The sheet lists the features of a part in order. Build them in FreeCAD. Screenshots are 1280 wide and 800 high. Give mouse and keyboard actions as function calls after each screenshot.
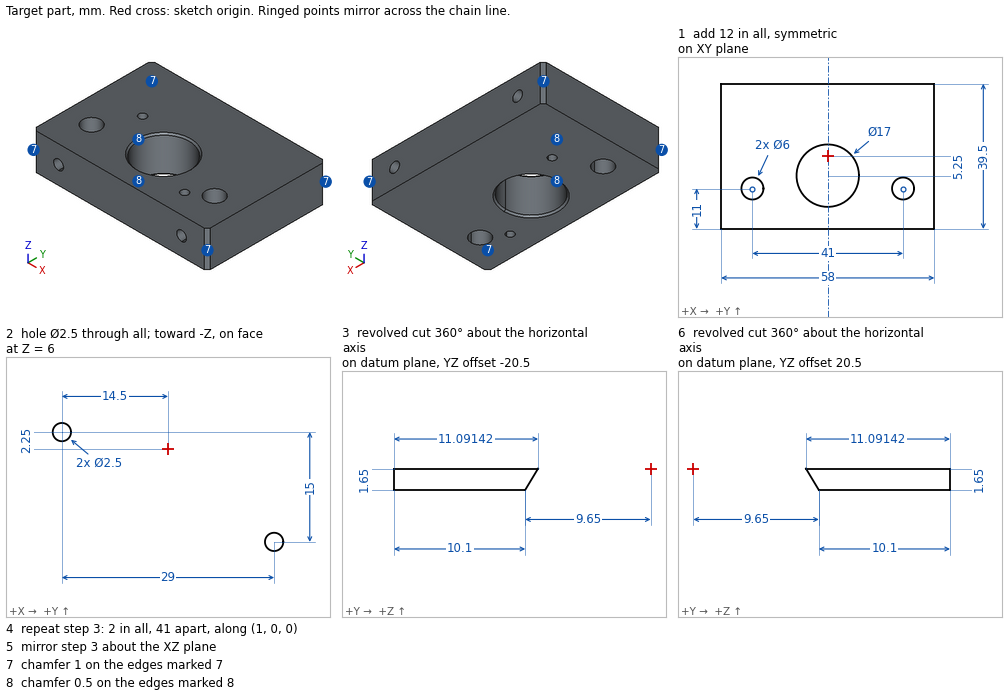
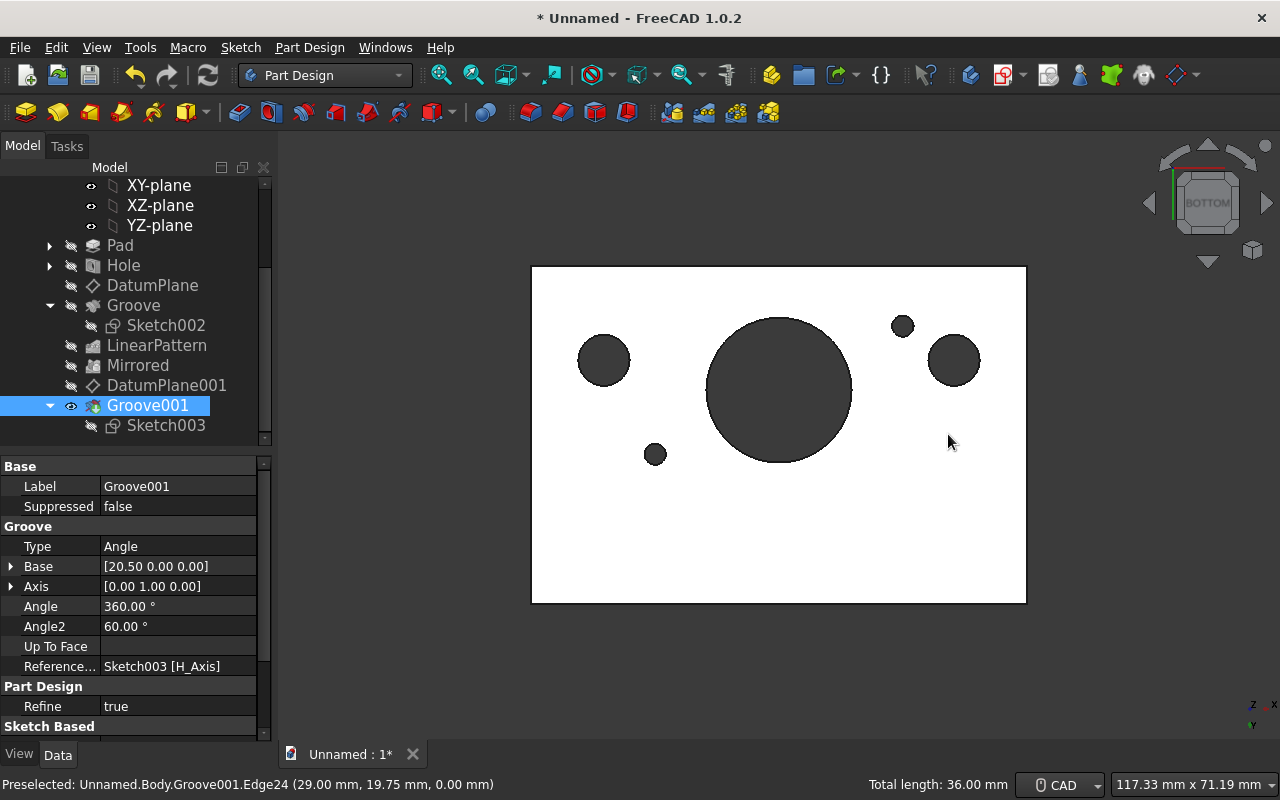
key(4)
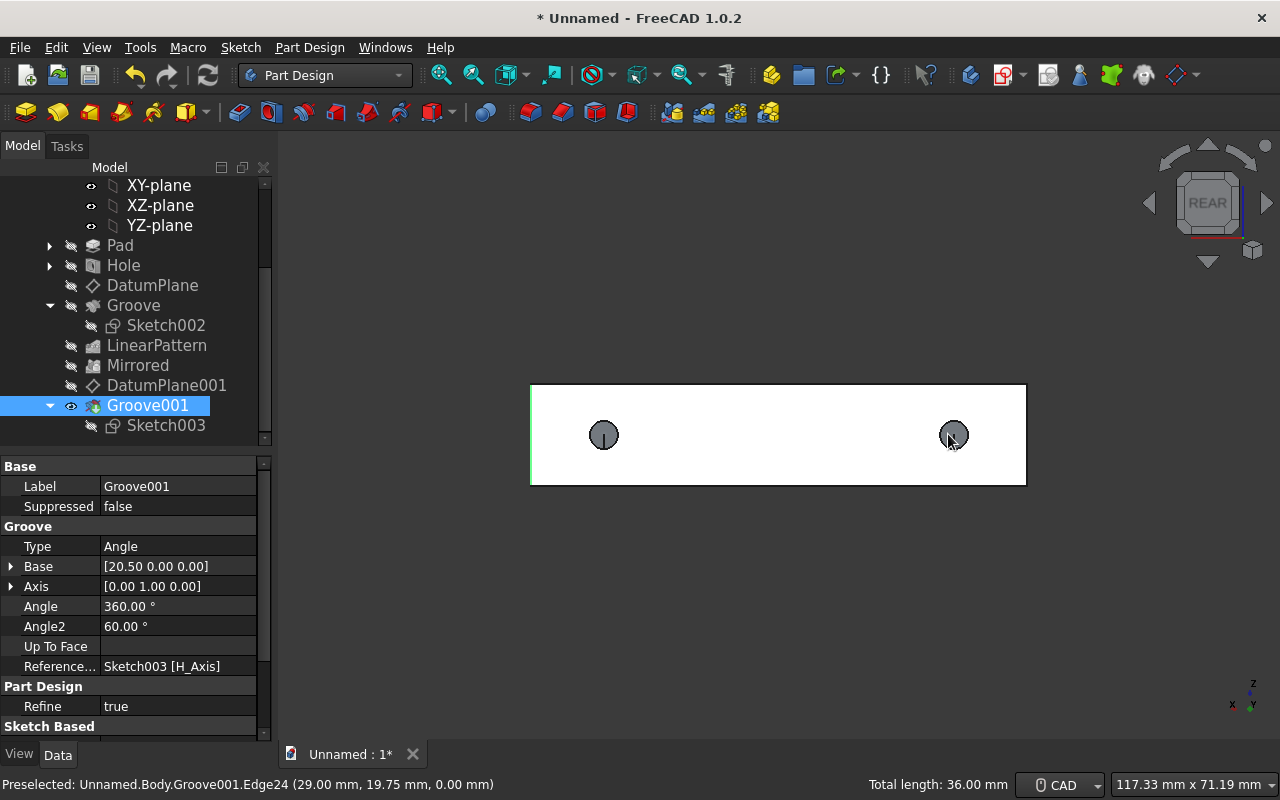
click(1027, 434, ctrl)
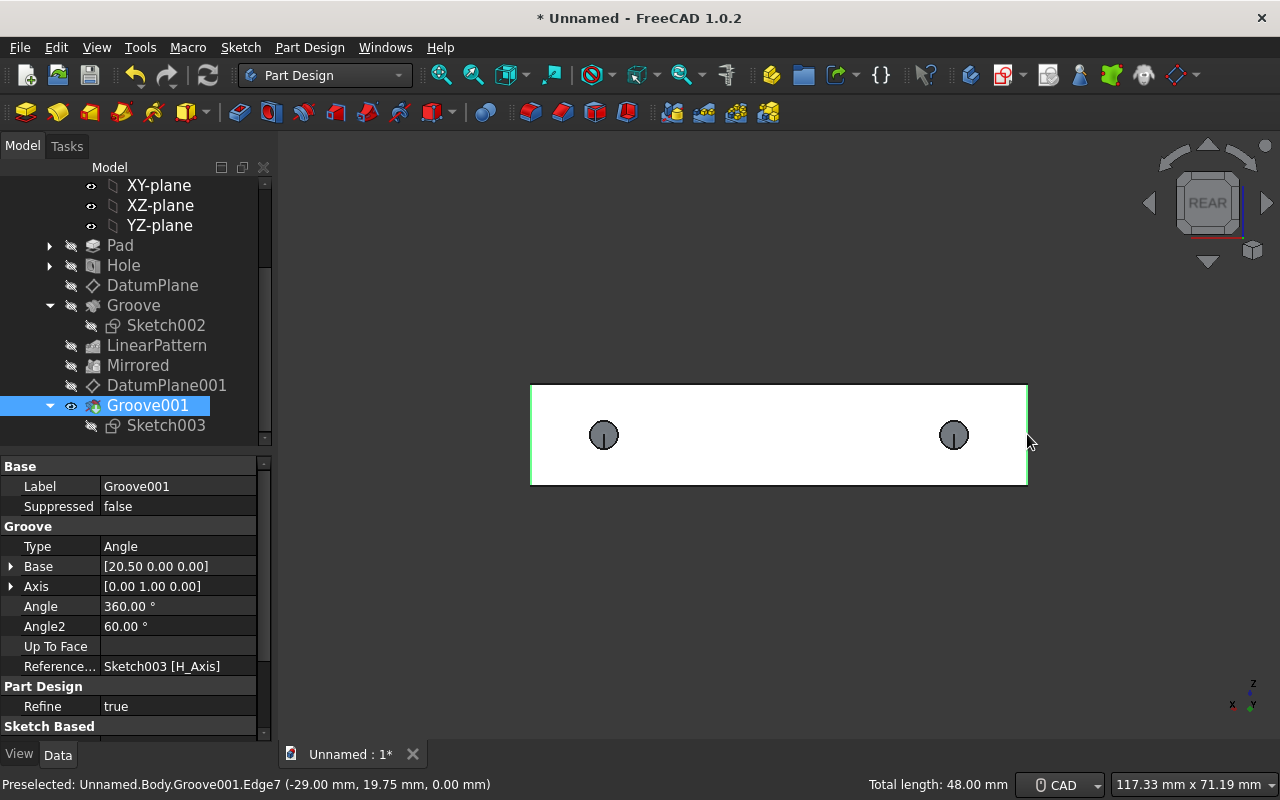
click(564, 112)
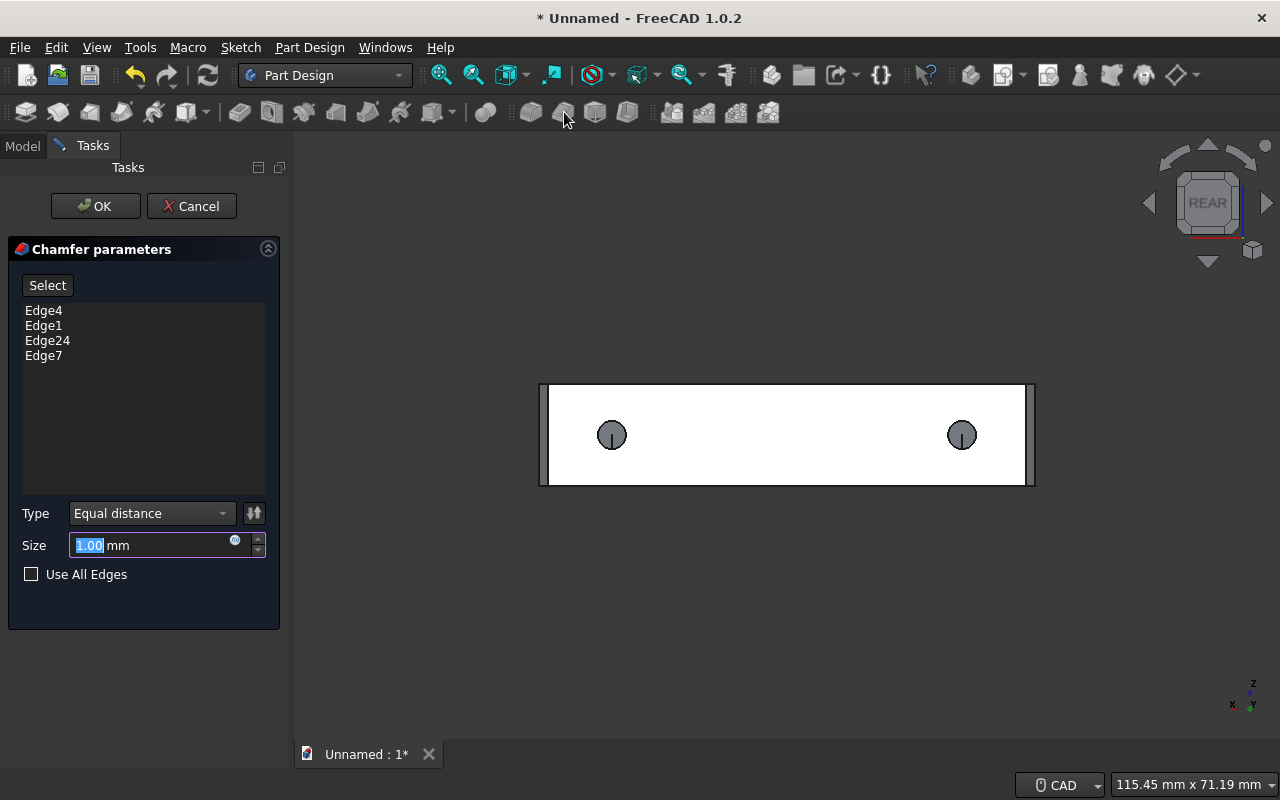
text(1)
key(Tab)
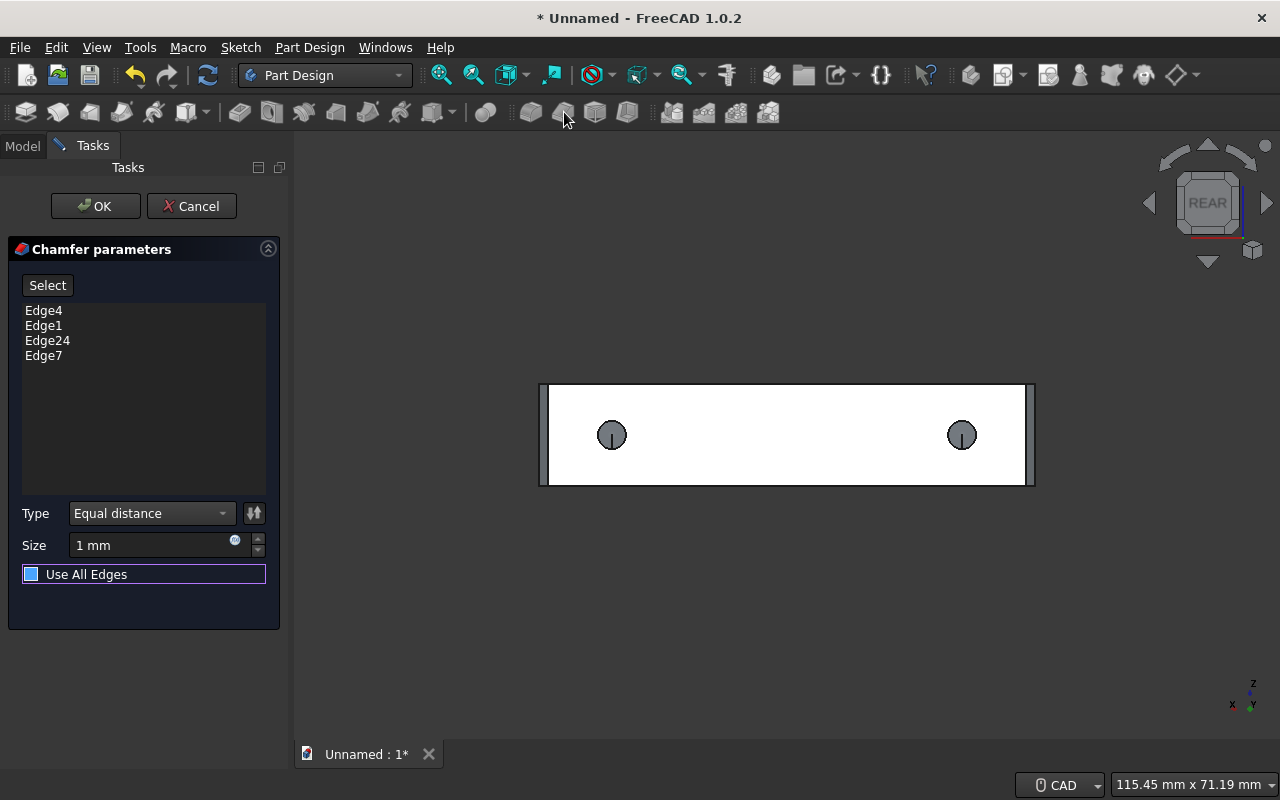
click(96, 206)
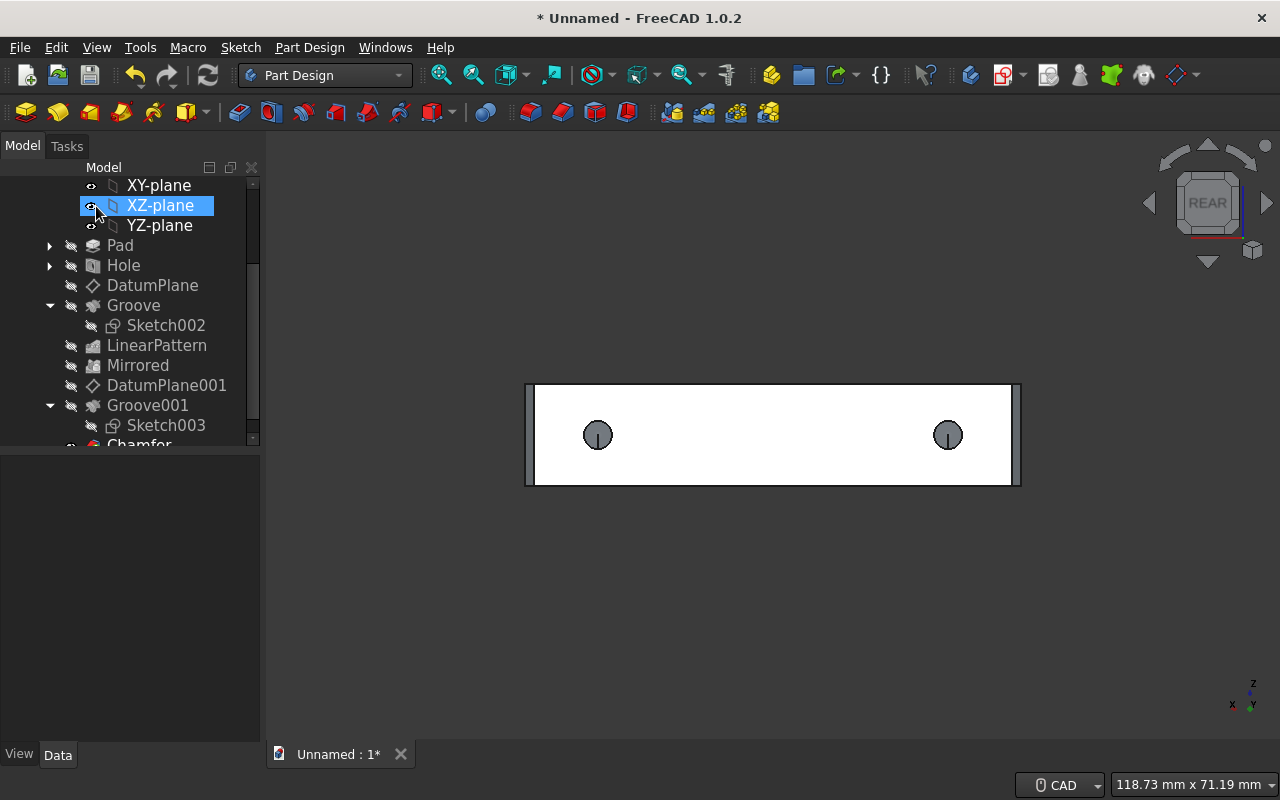
key(0)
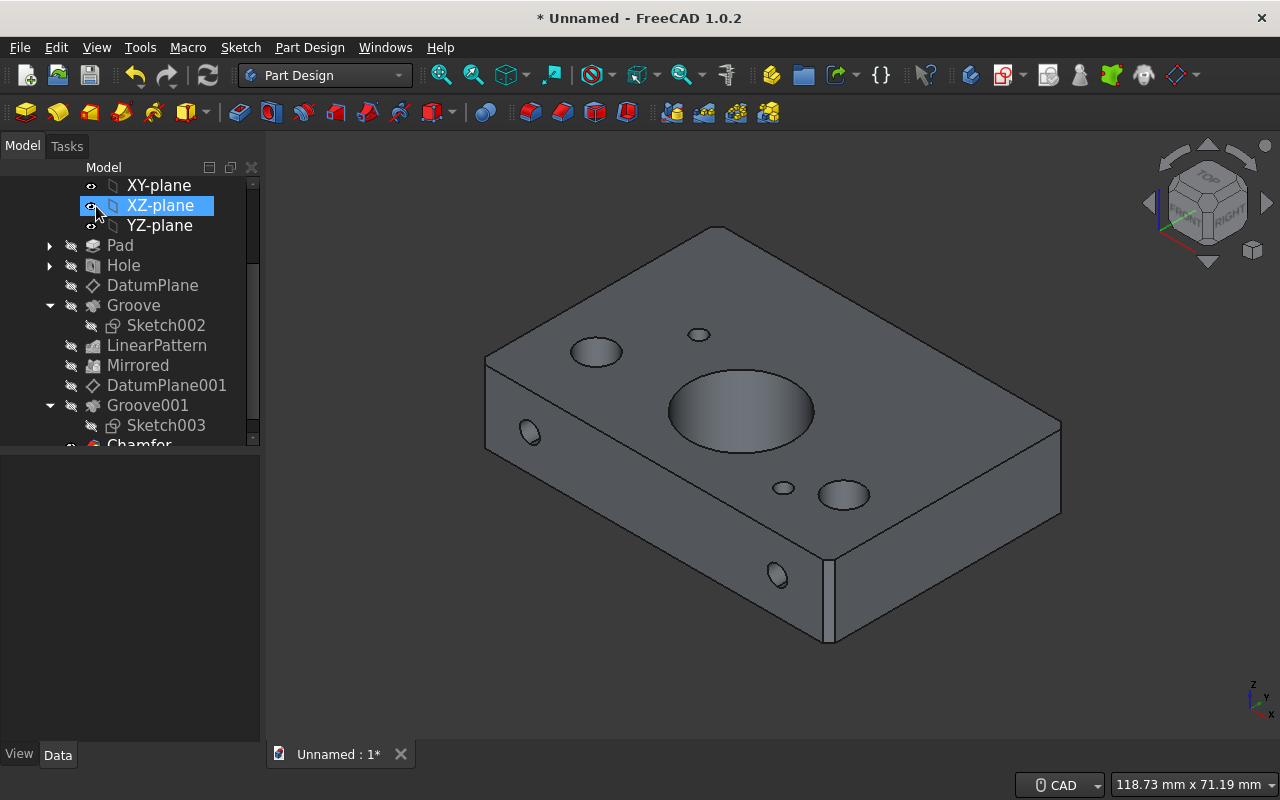
click(690, 381)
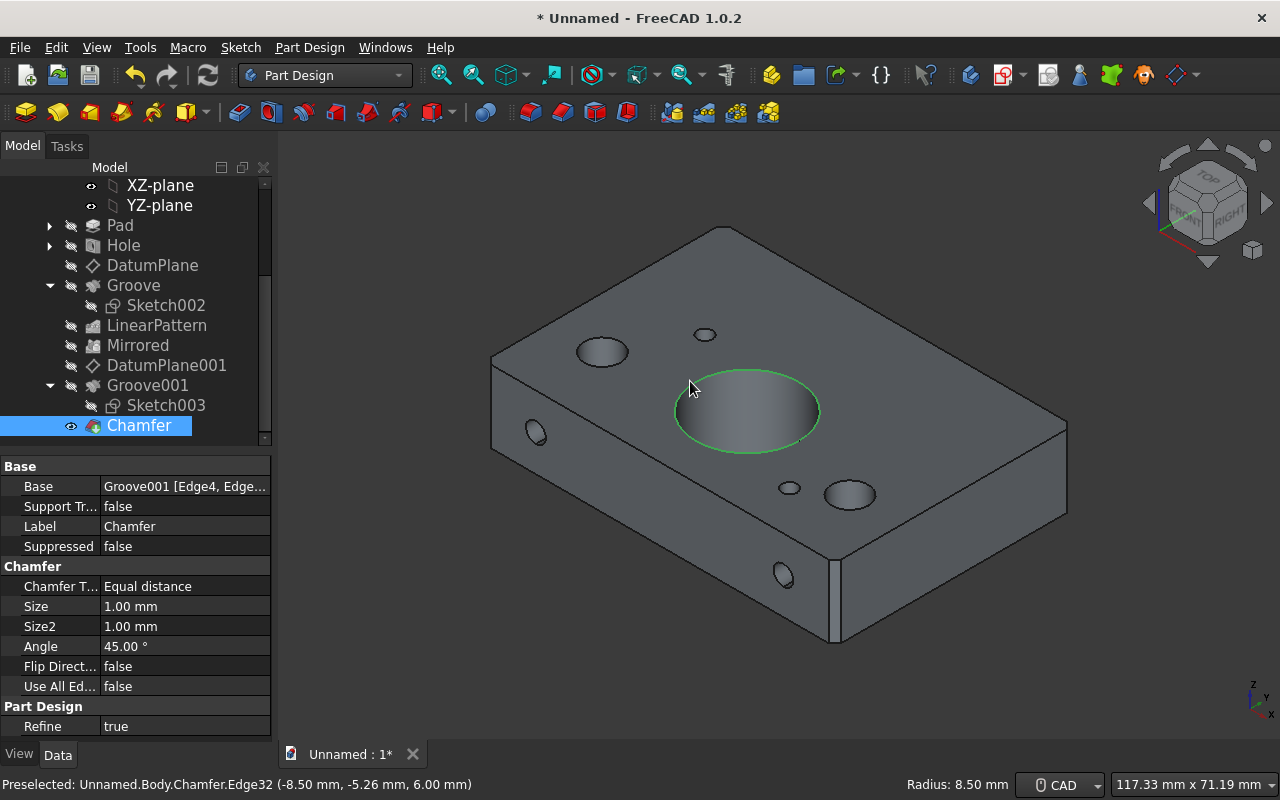
key(2)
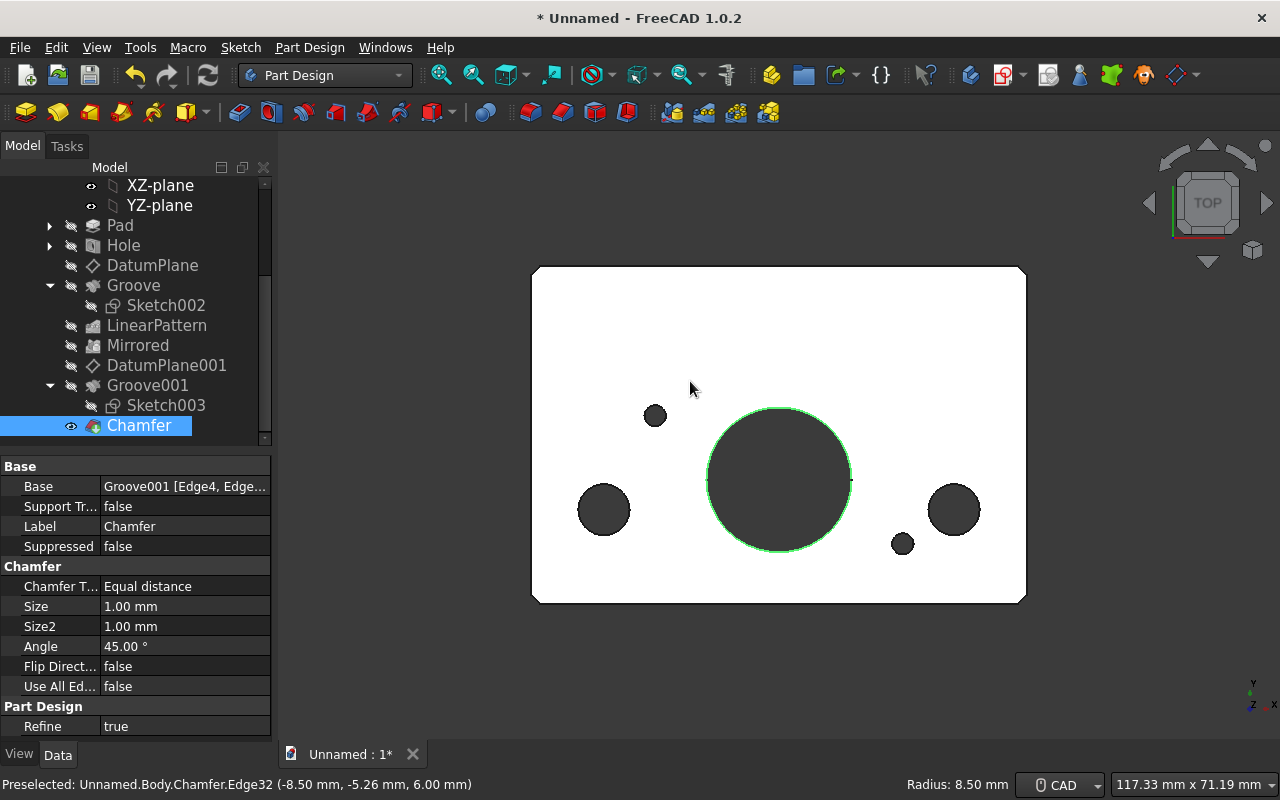
key(1)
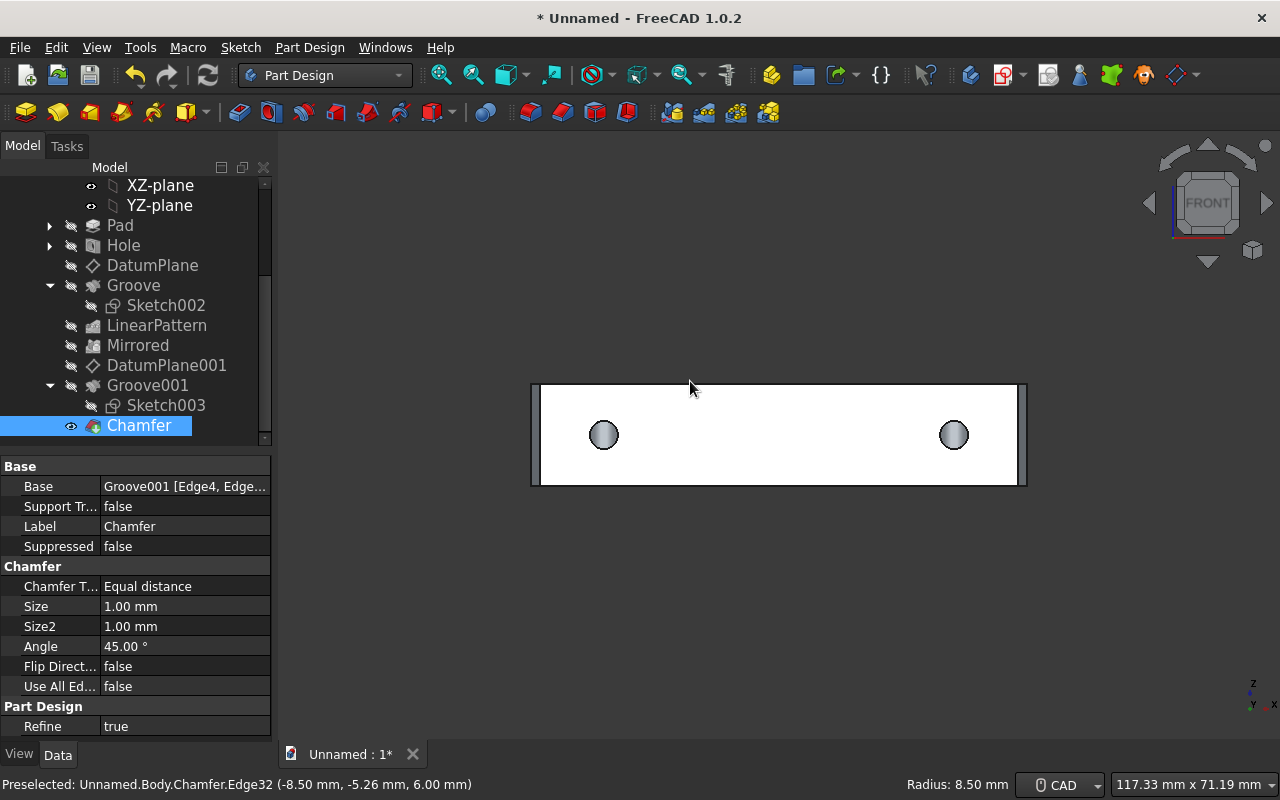
key(3)